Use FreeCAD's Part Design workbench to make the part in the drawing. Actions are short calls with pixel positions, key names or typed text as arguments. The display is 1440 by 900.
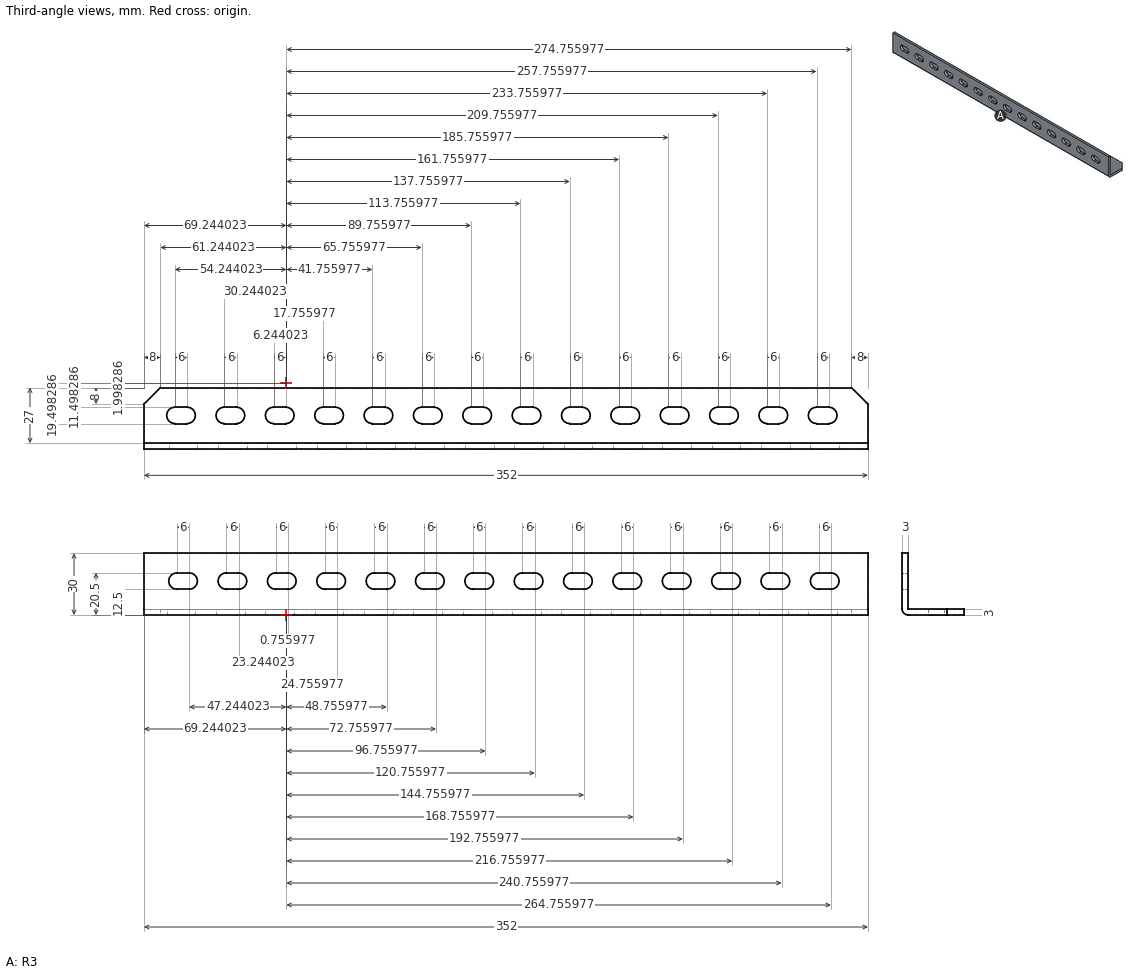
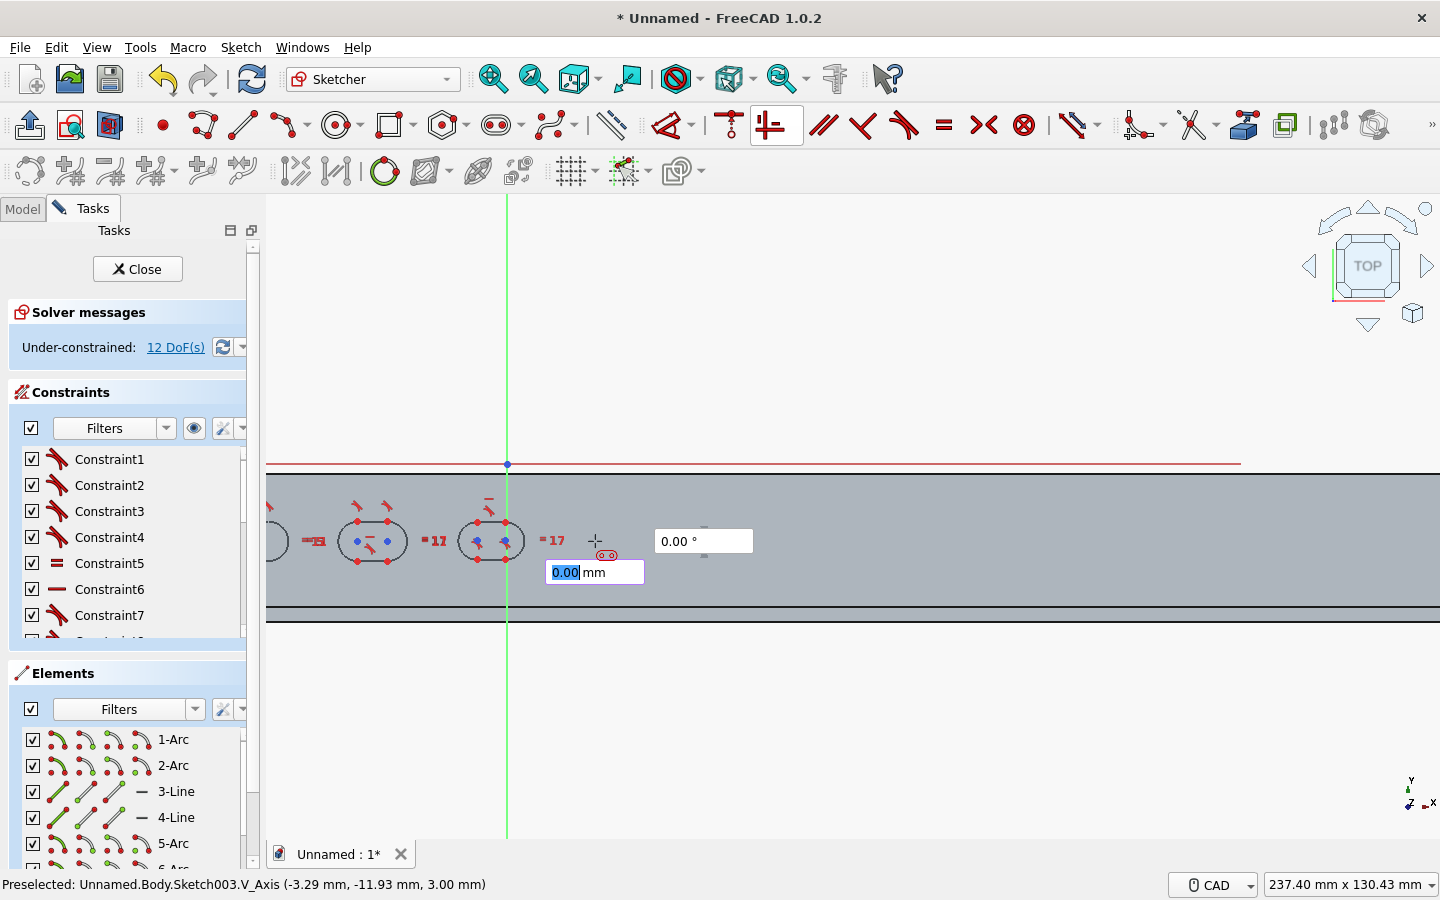
click(625, 541)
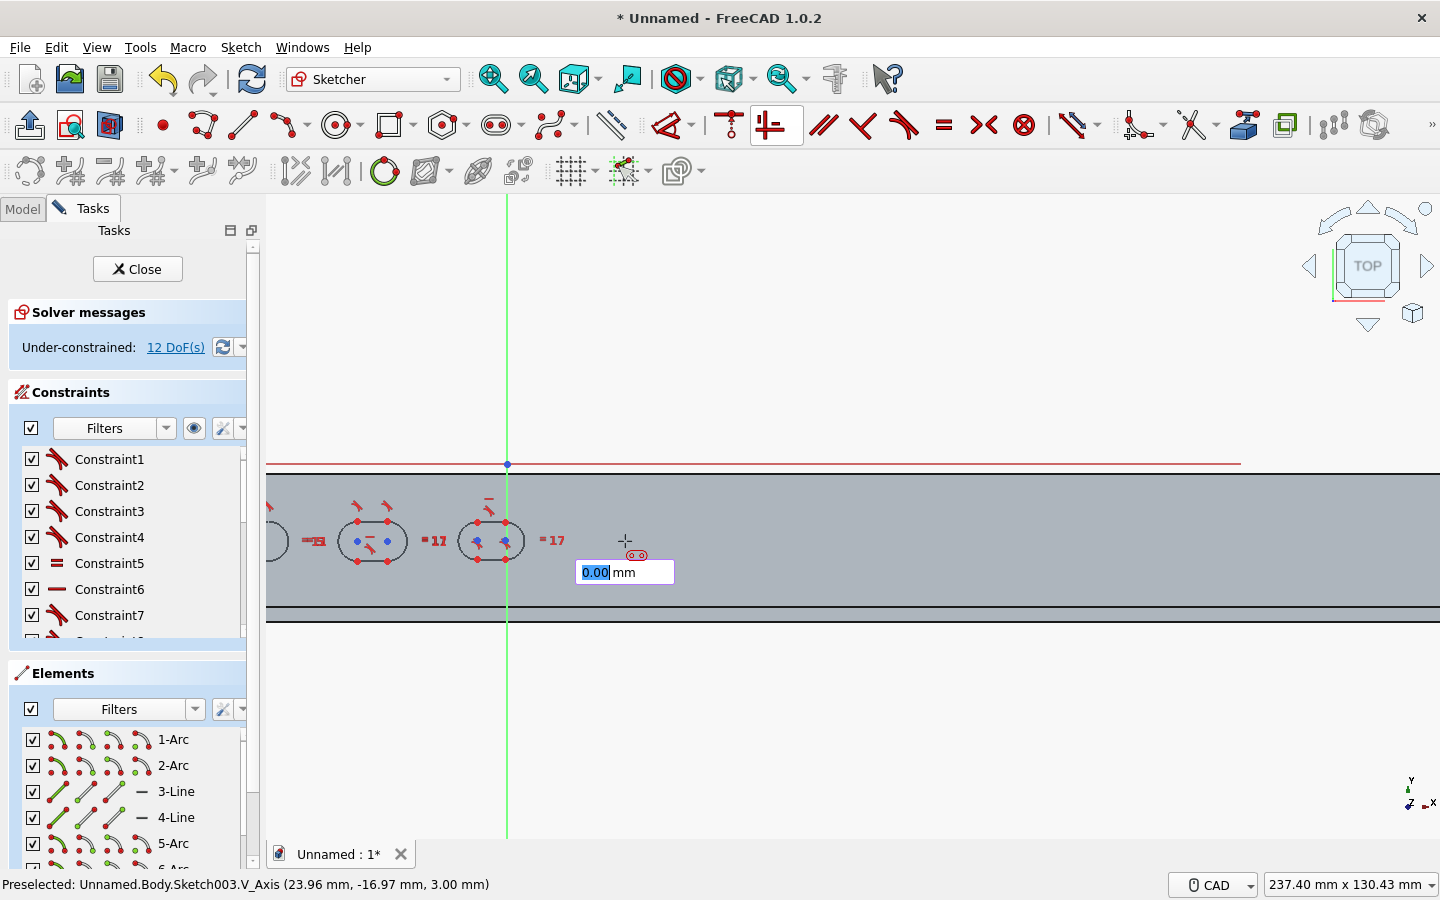
click(610, 521)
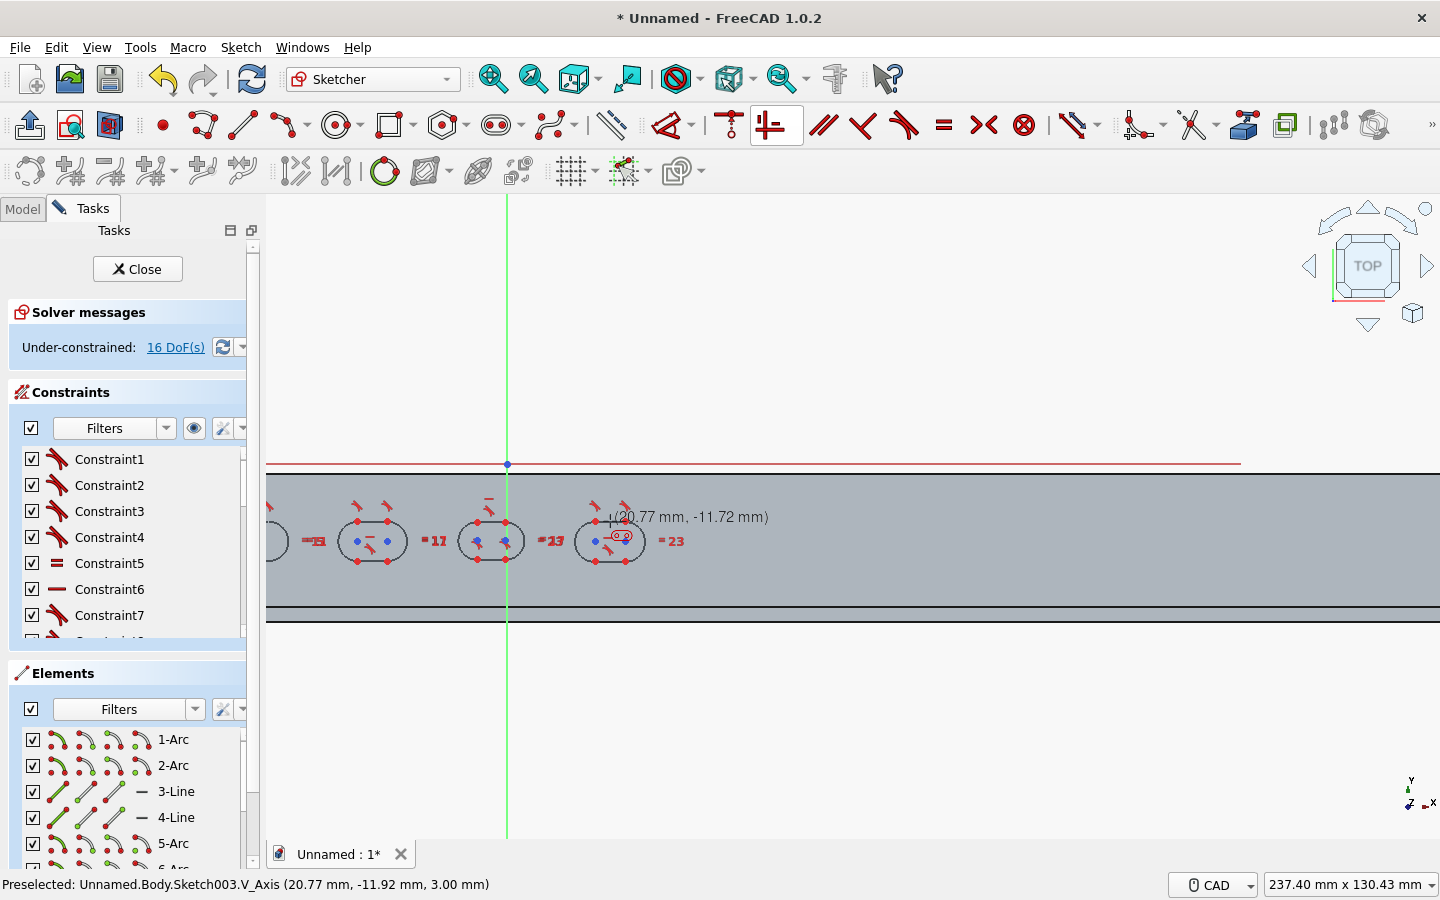
click(714, 541)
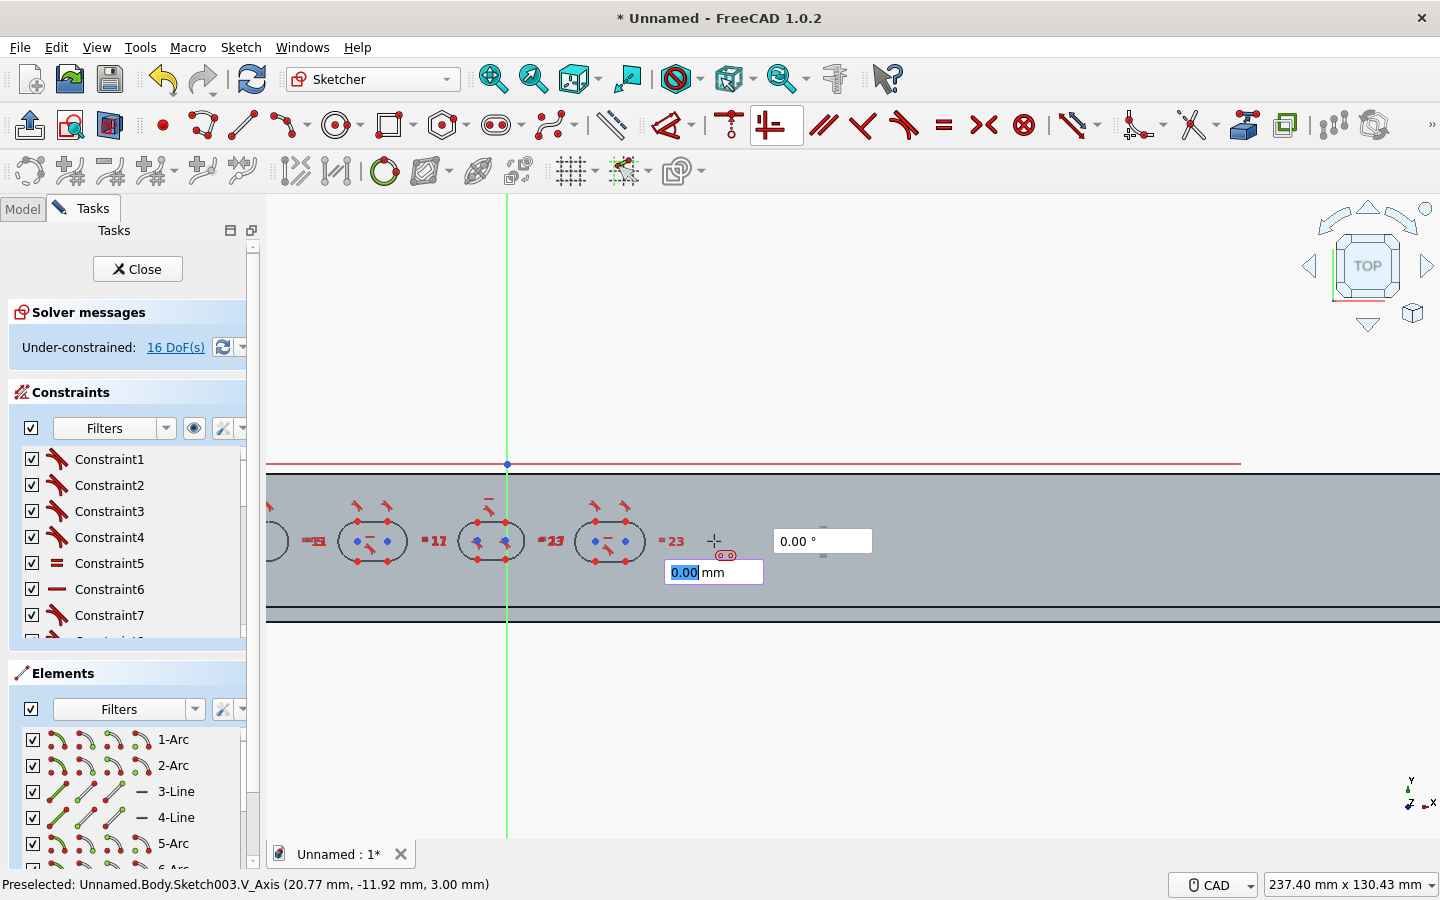
click(743, 541)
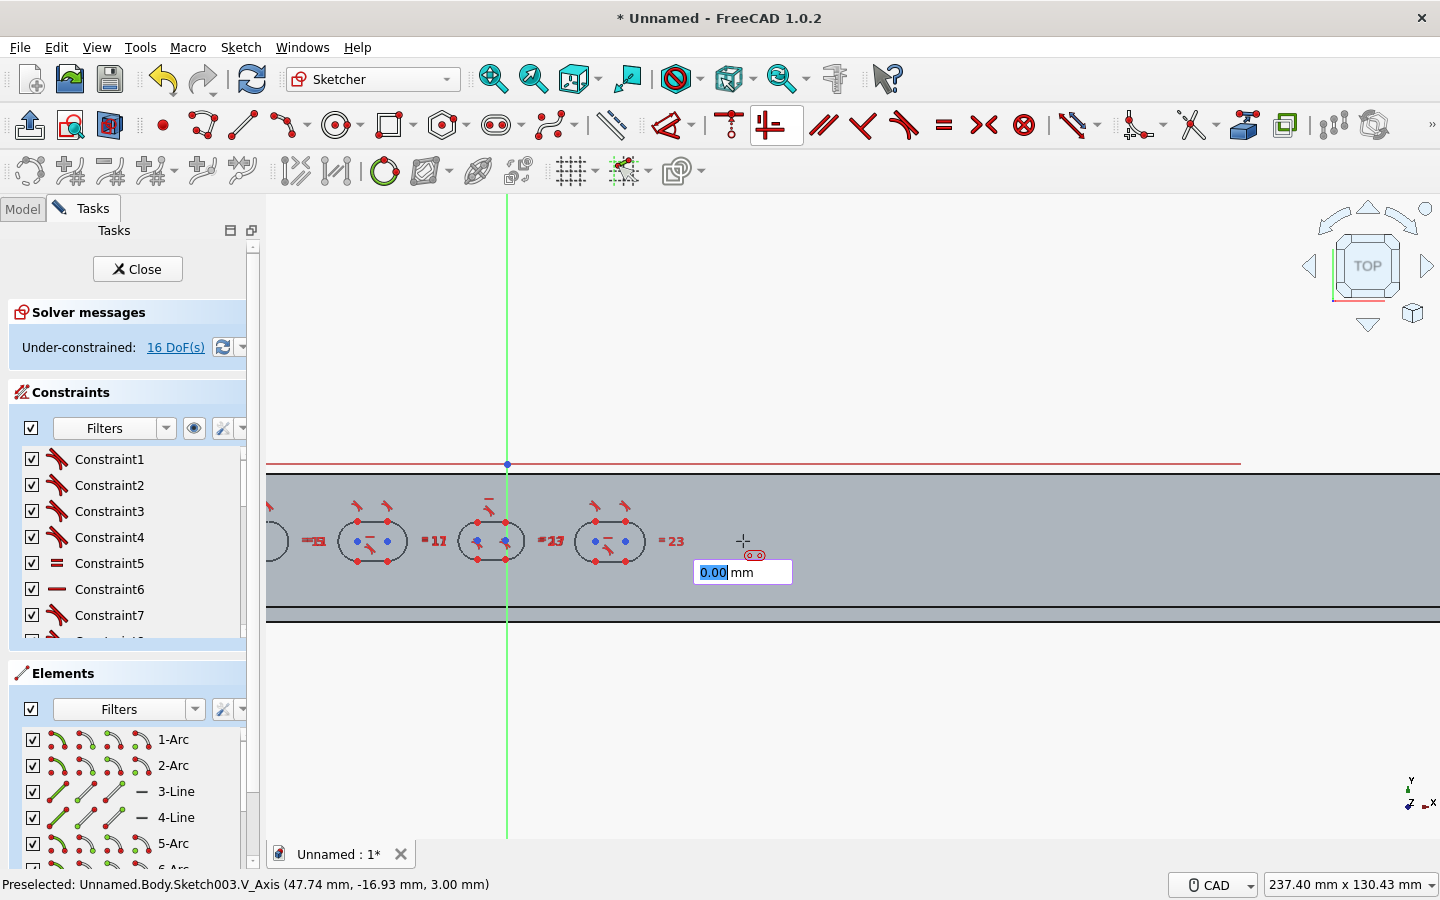
click(729, 521)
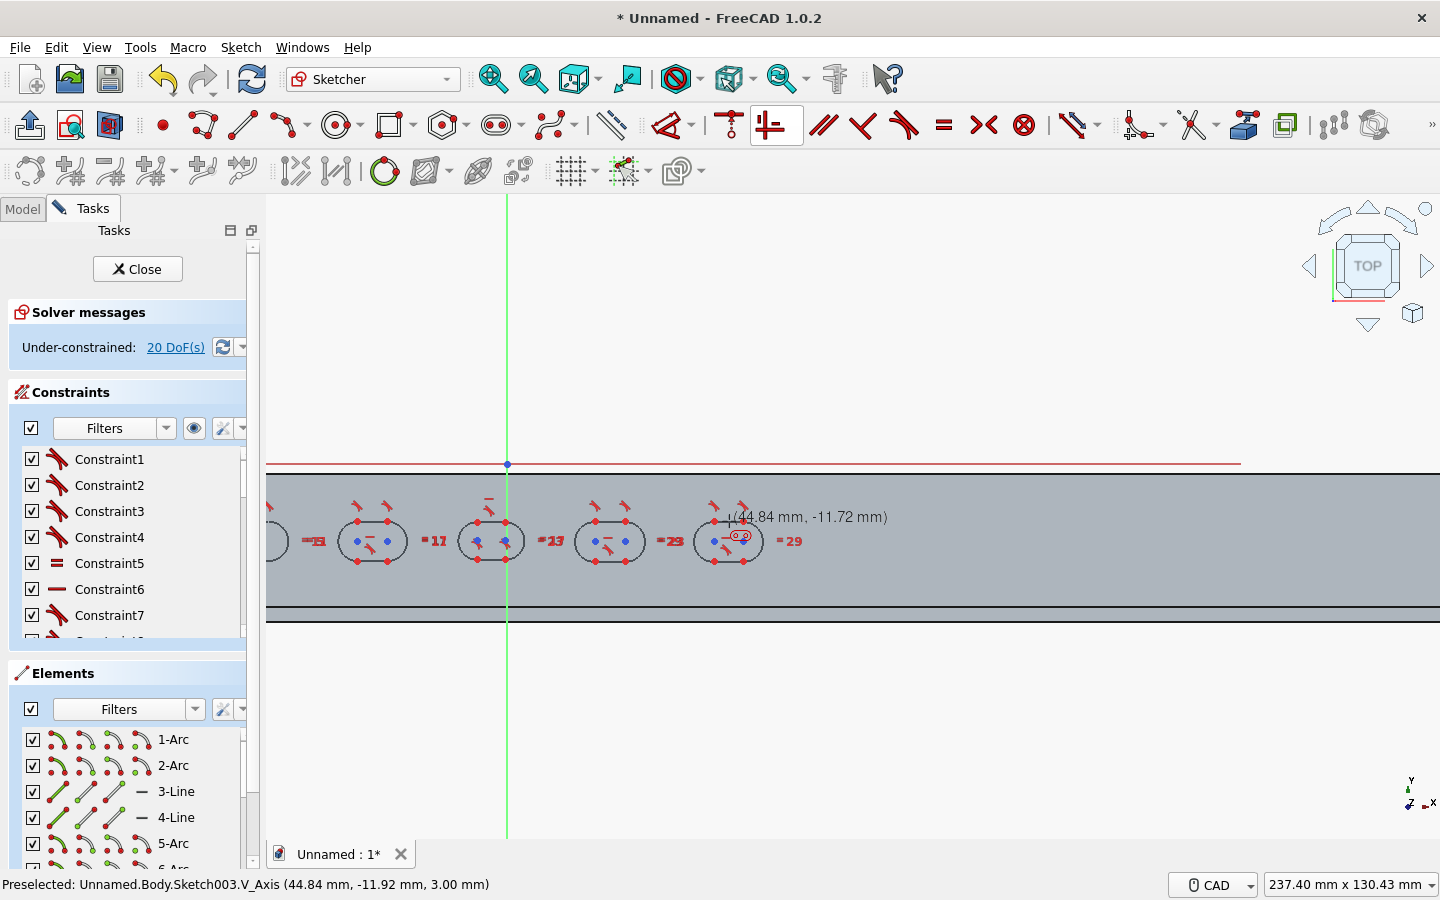
click(832, 541)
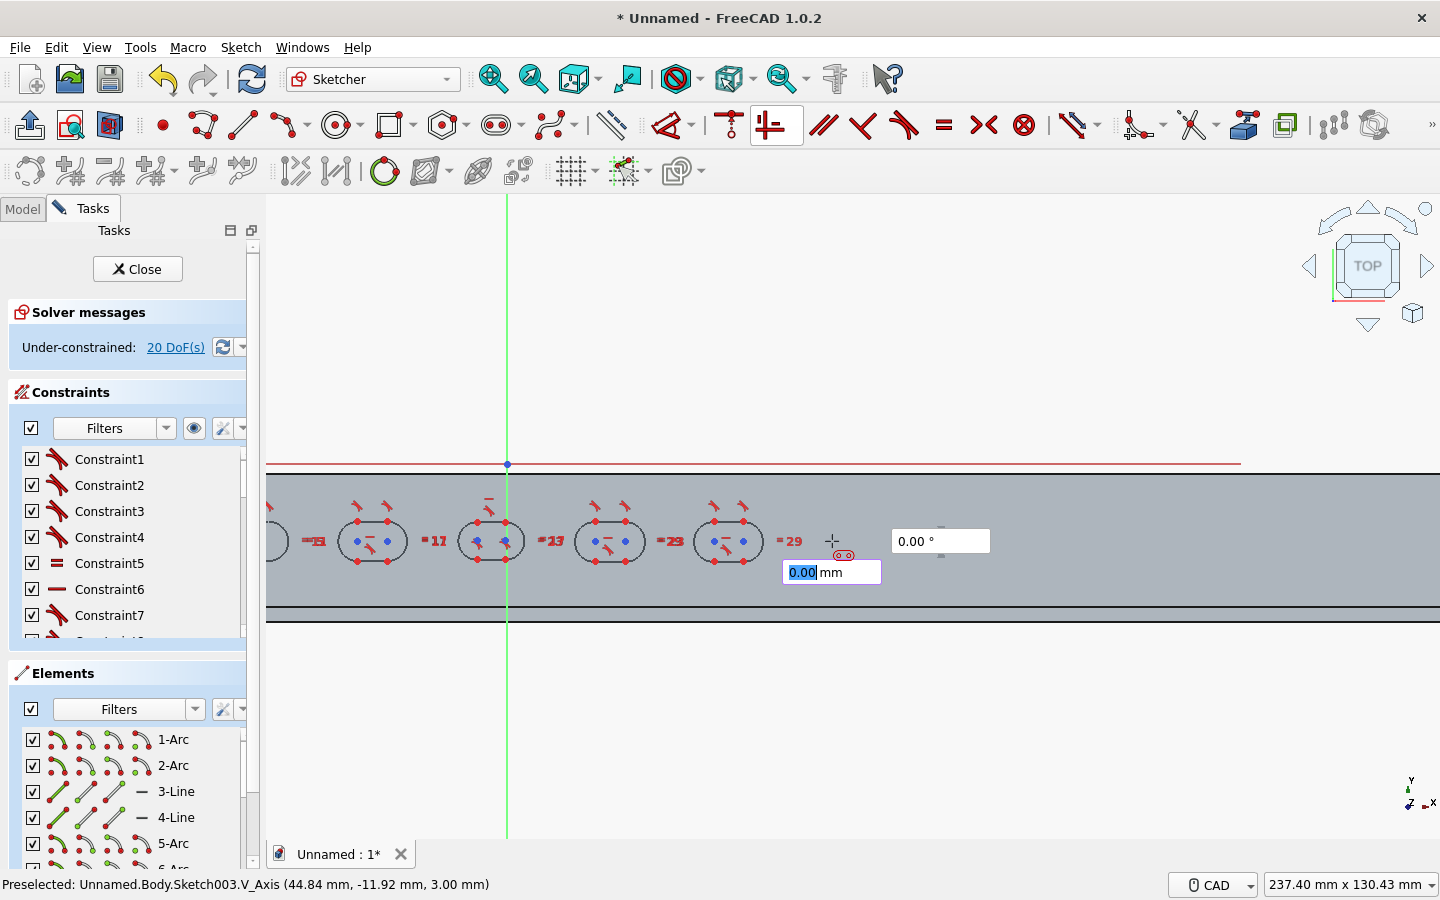
click(862, 541)